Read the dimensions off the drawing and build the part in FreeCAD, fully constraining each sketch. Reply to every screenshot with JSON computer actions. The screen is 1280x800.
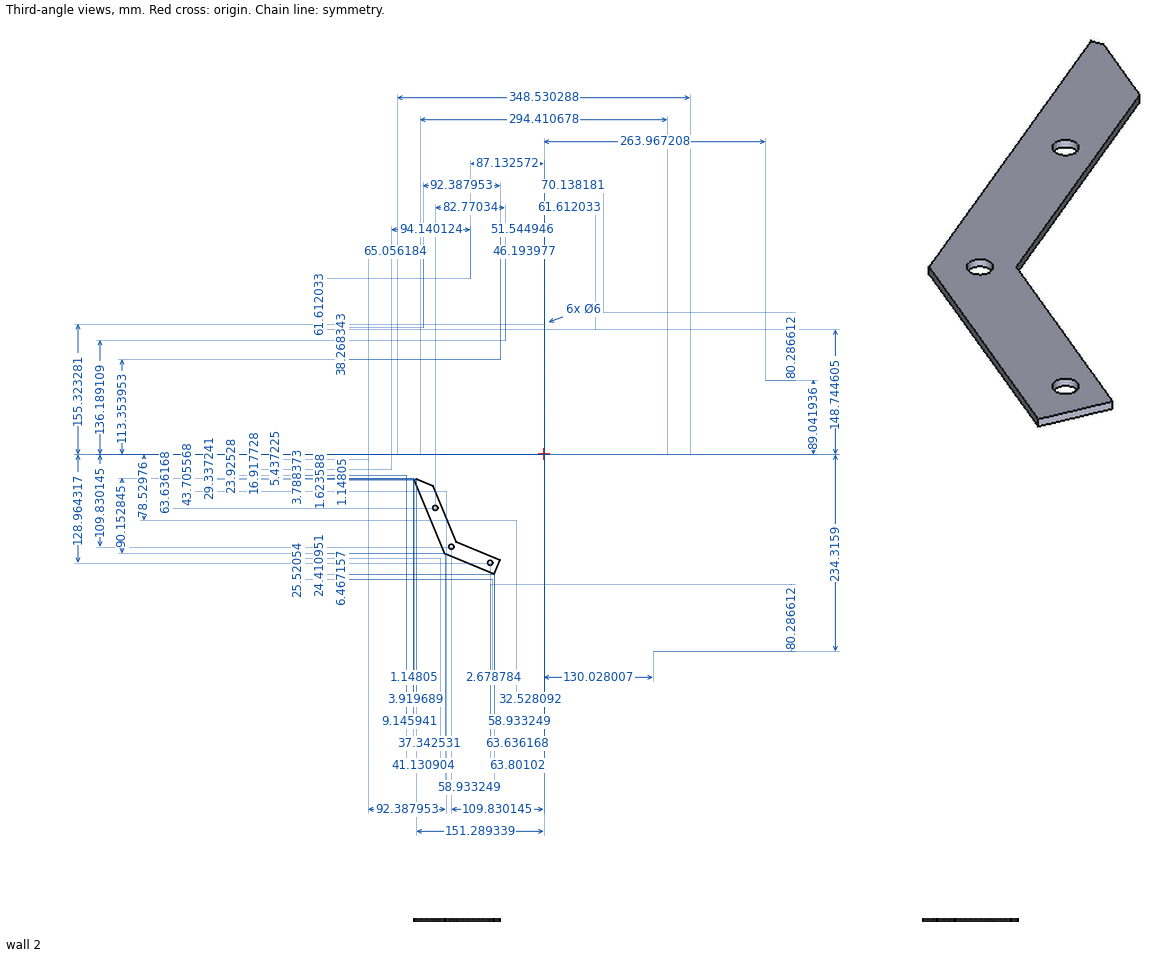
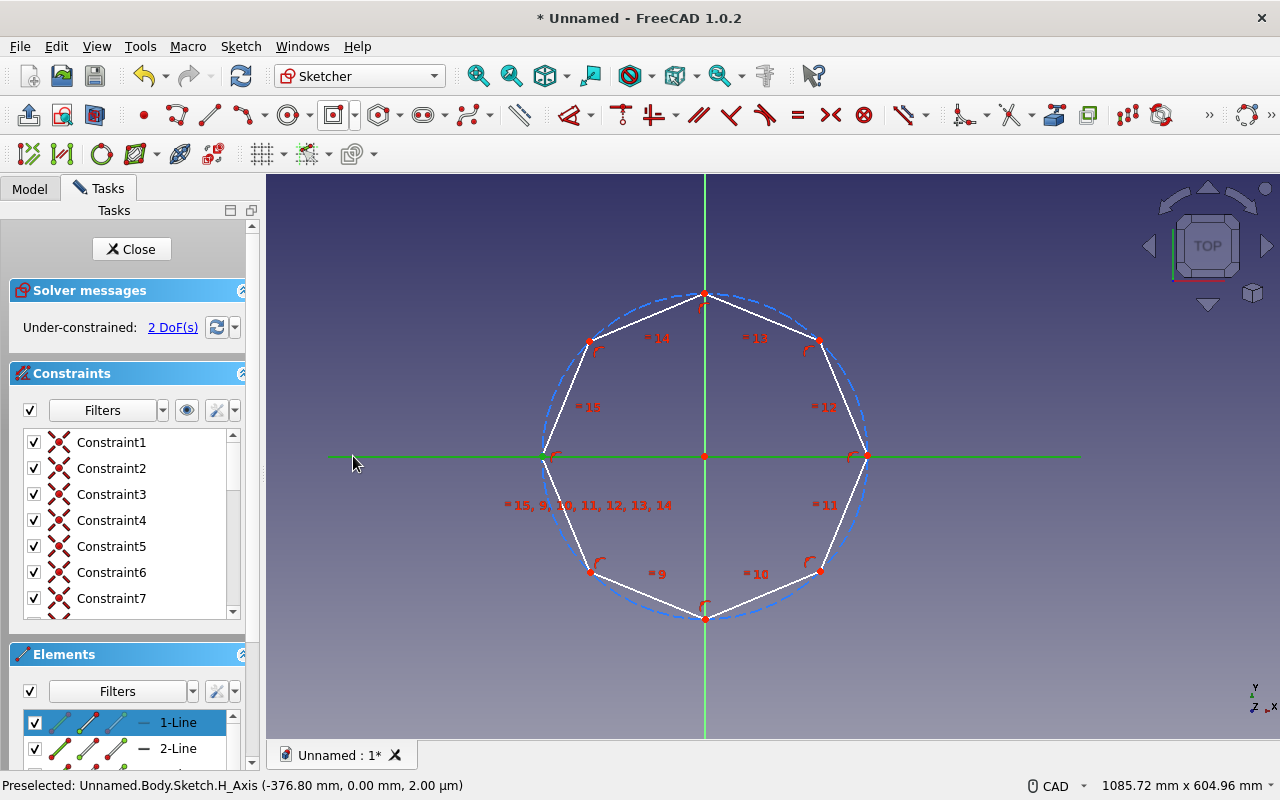
{"action": "left_click", "coordinate": [621, 116]}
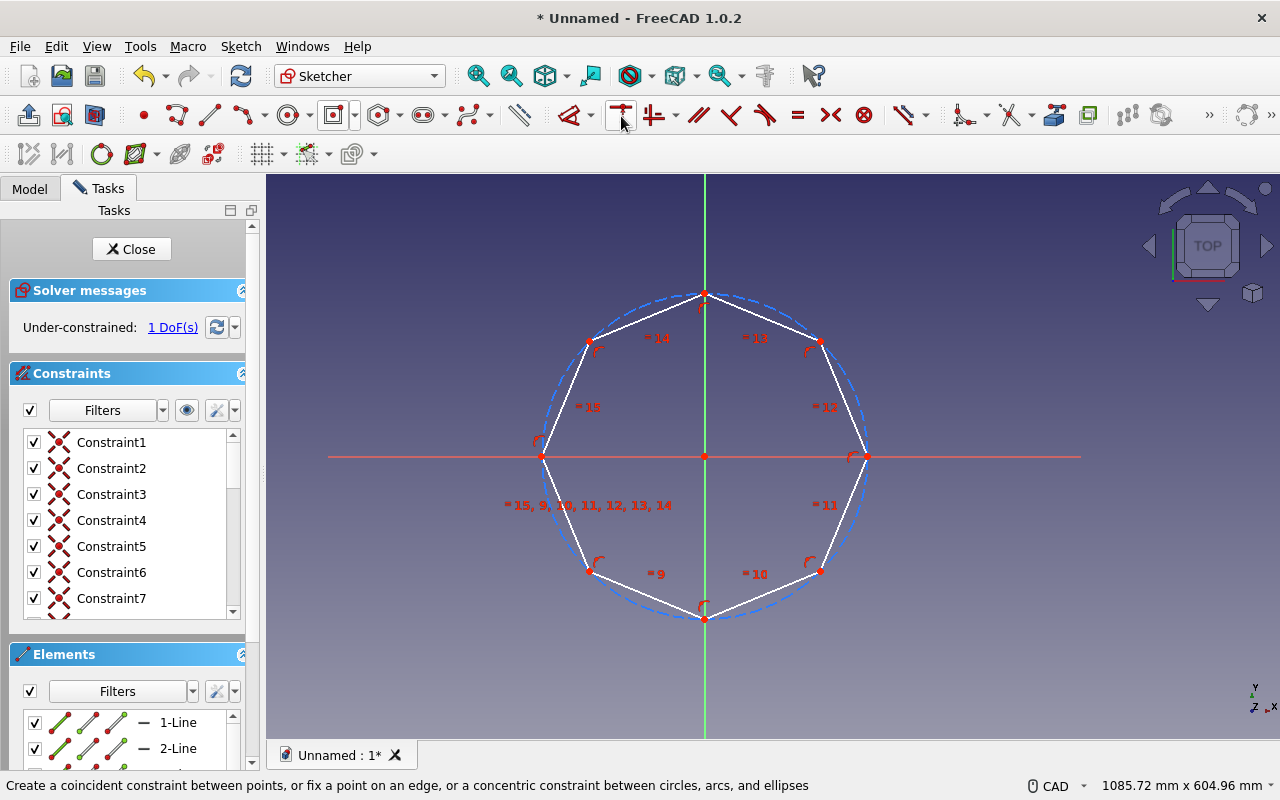
{"action": "left_click", "coordinate": [568, 116]}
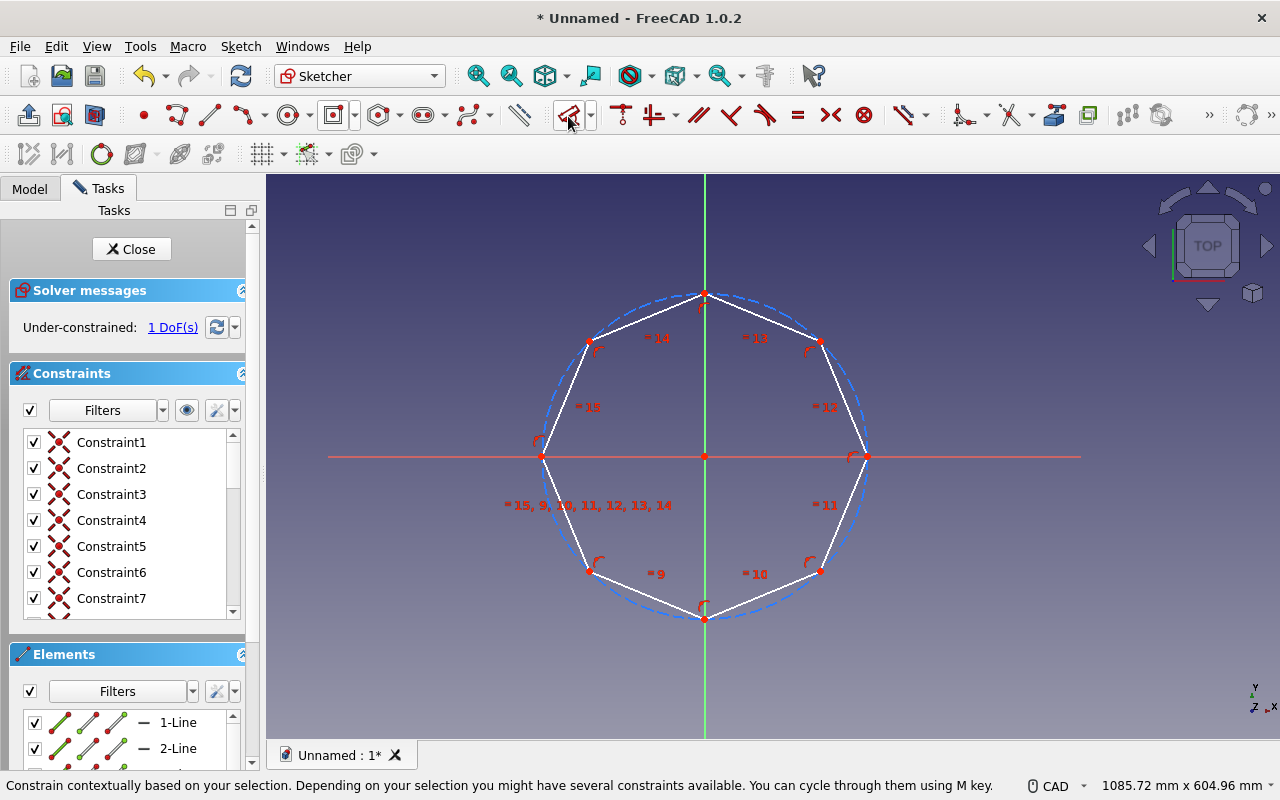
{"action": "left_click", "coordinate": [542, 456]}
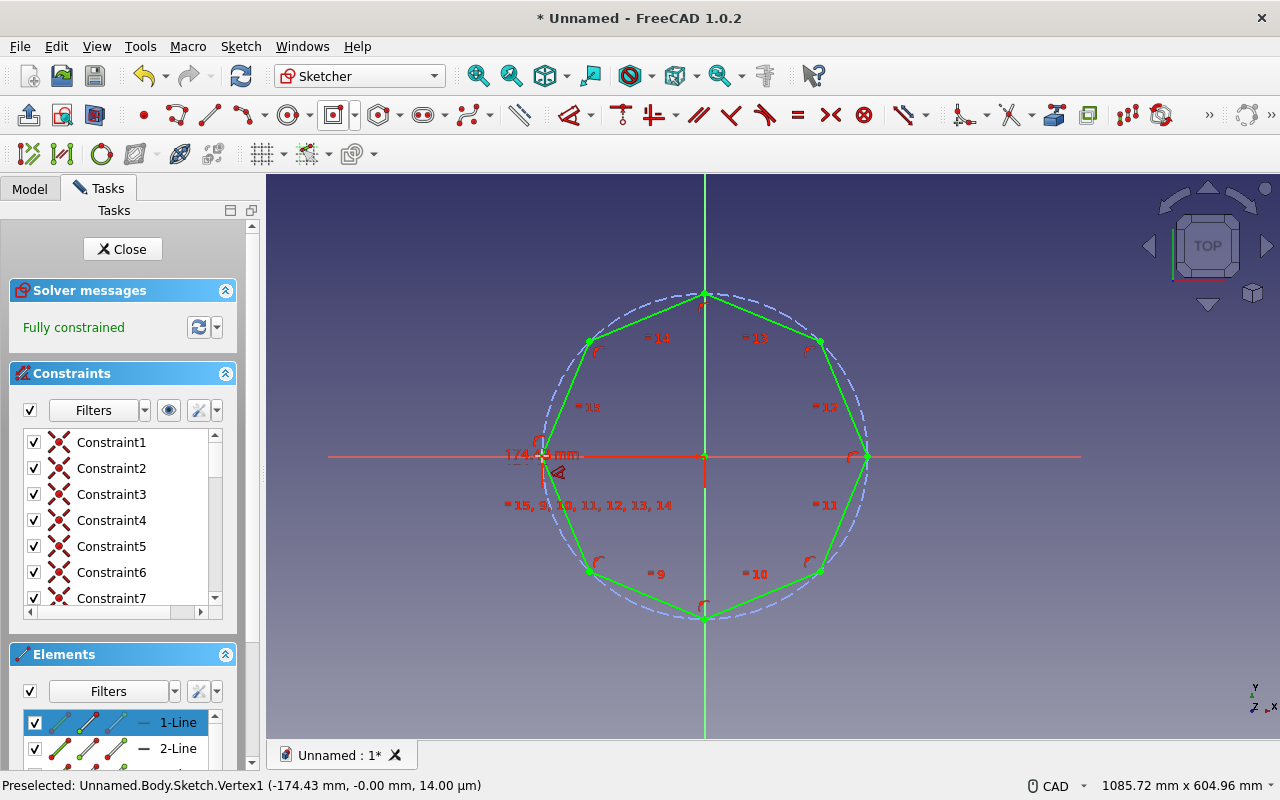
{"action": "left_click", "coordinate": [868, 457]}
{"action": "left_click", "coordinate": [630, 491]}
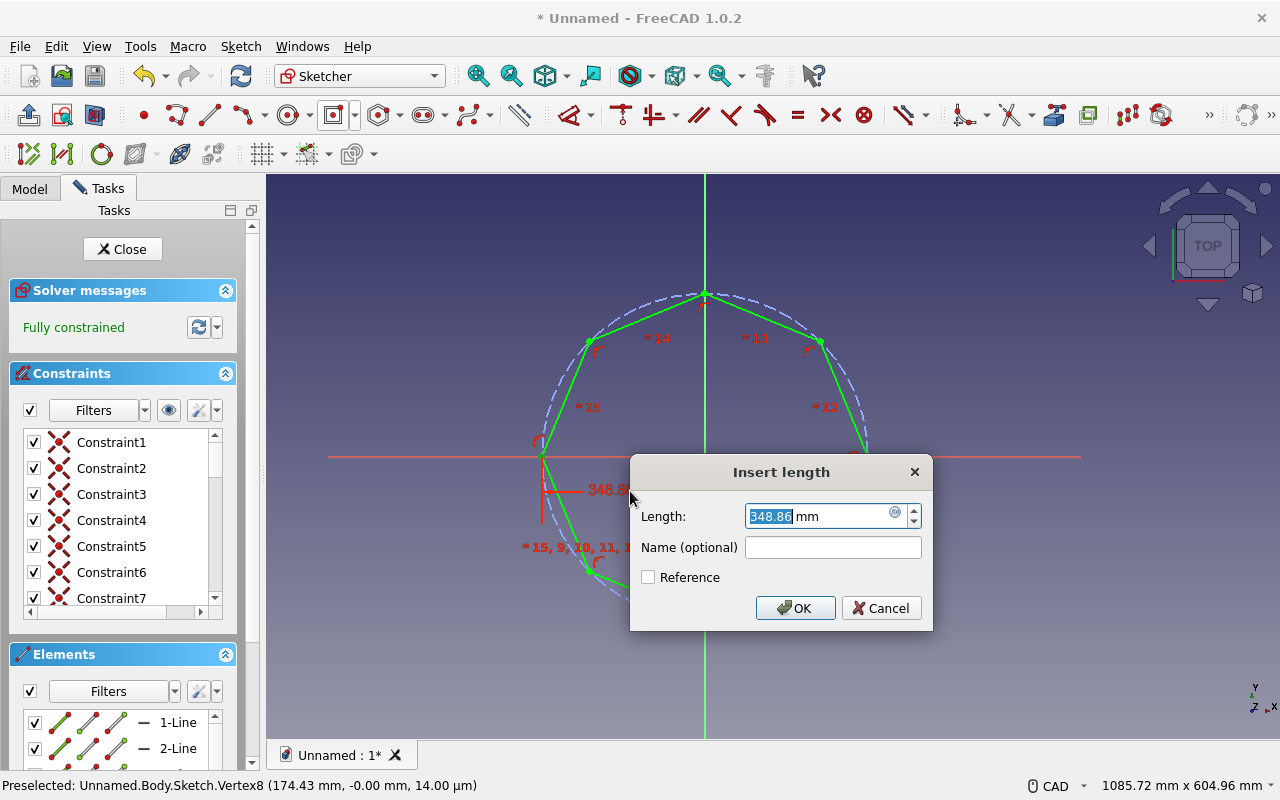
{"action": "type", "text": "348.530288"}
{"action": "key", "text": "Return"}
{"action": "key", "text": "Escape"}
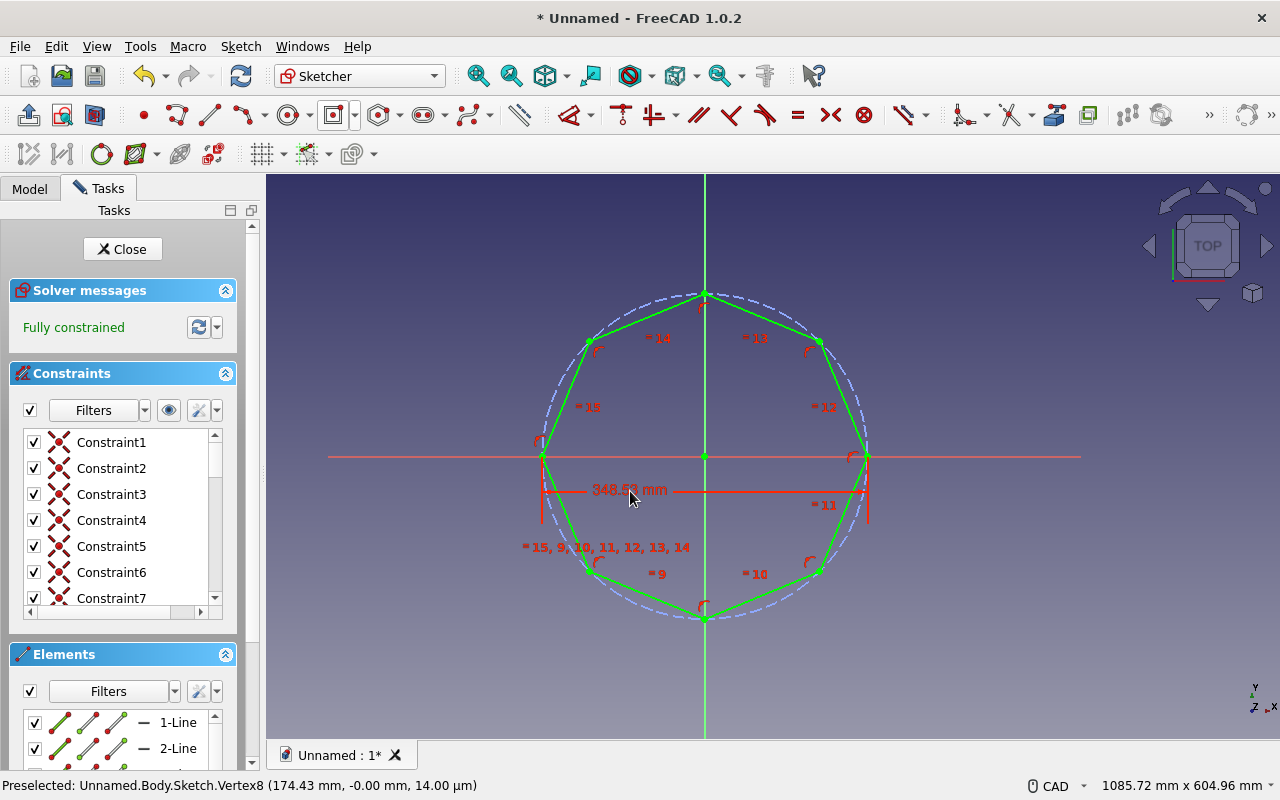
{"action": "left_click", "coordinate": [123, 249]}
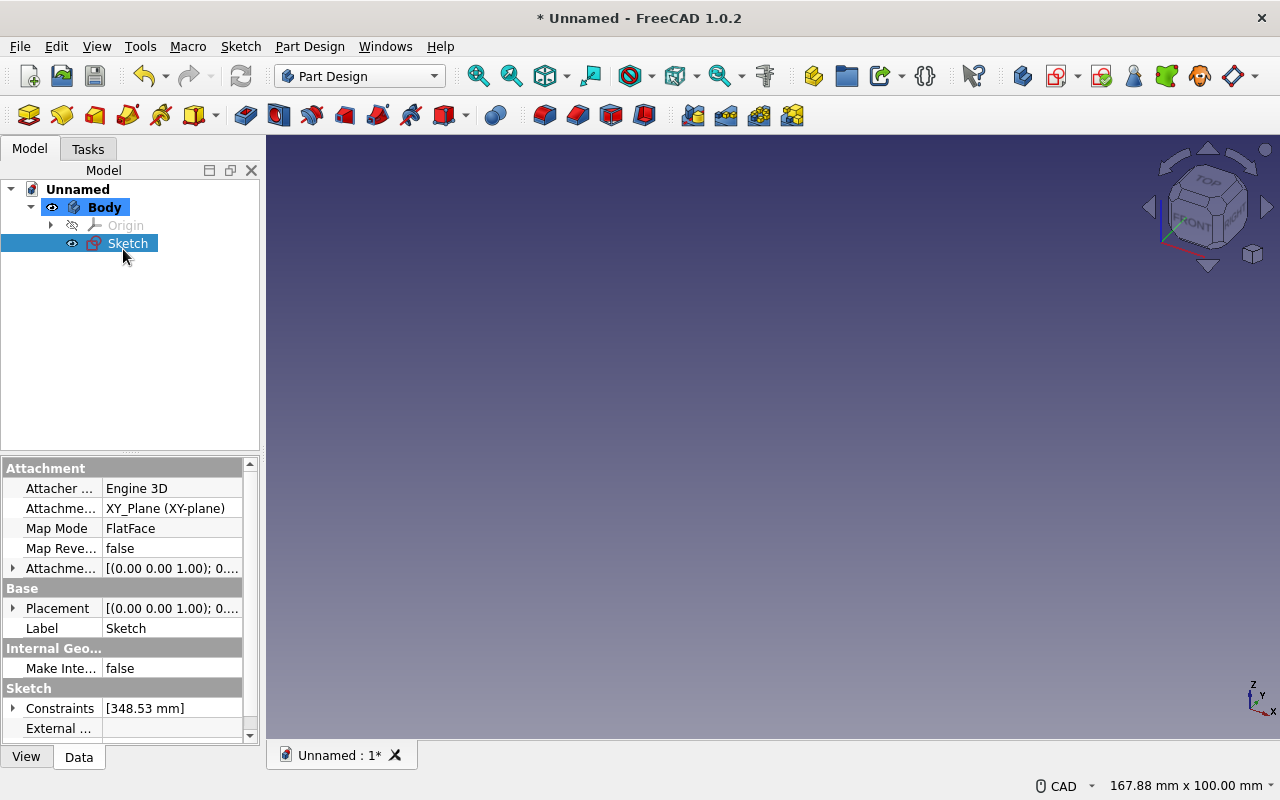
{"action": "left_click", "coordinate": [29, 116]}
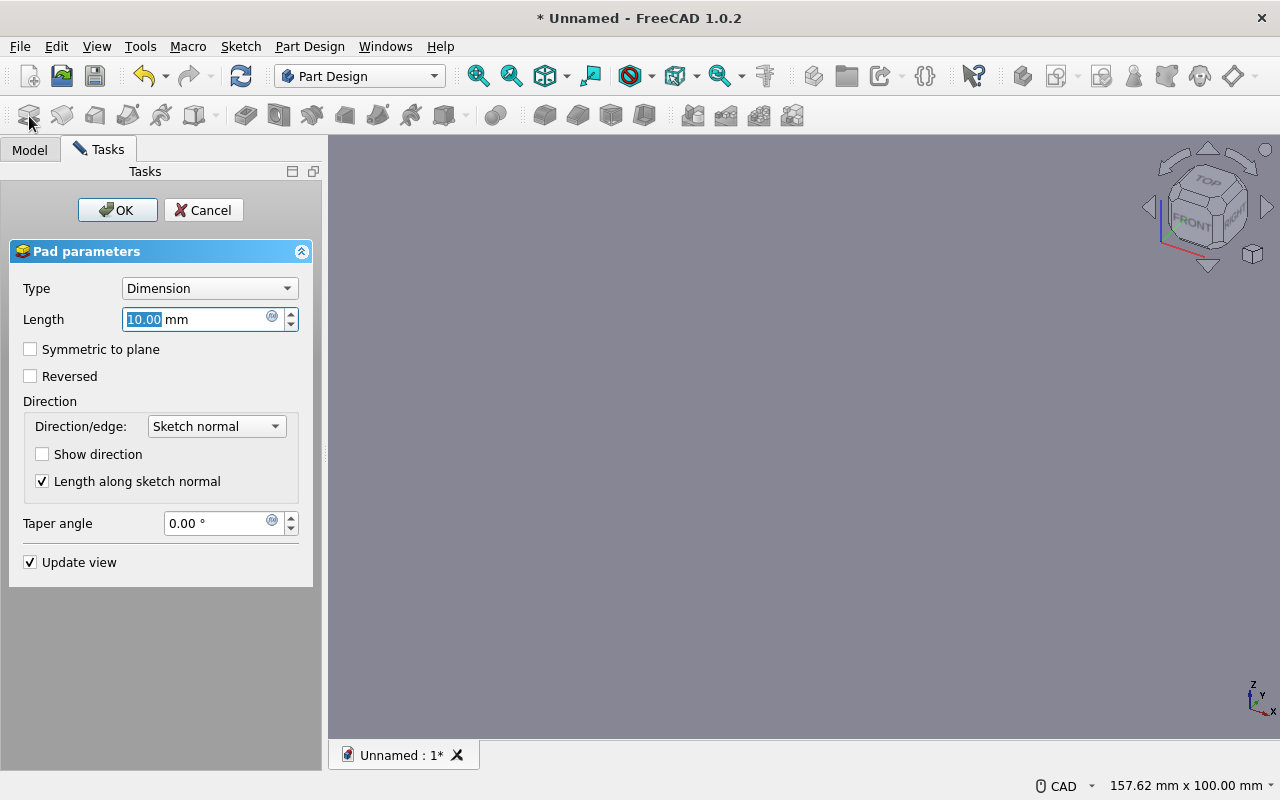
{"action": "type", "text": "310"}
{"action": "key", "text": "Tab"}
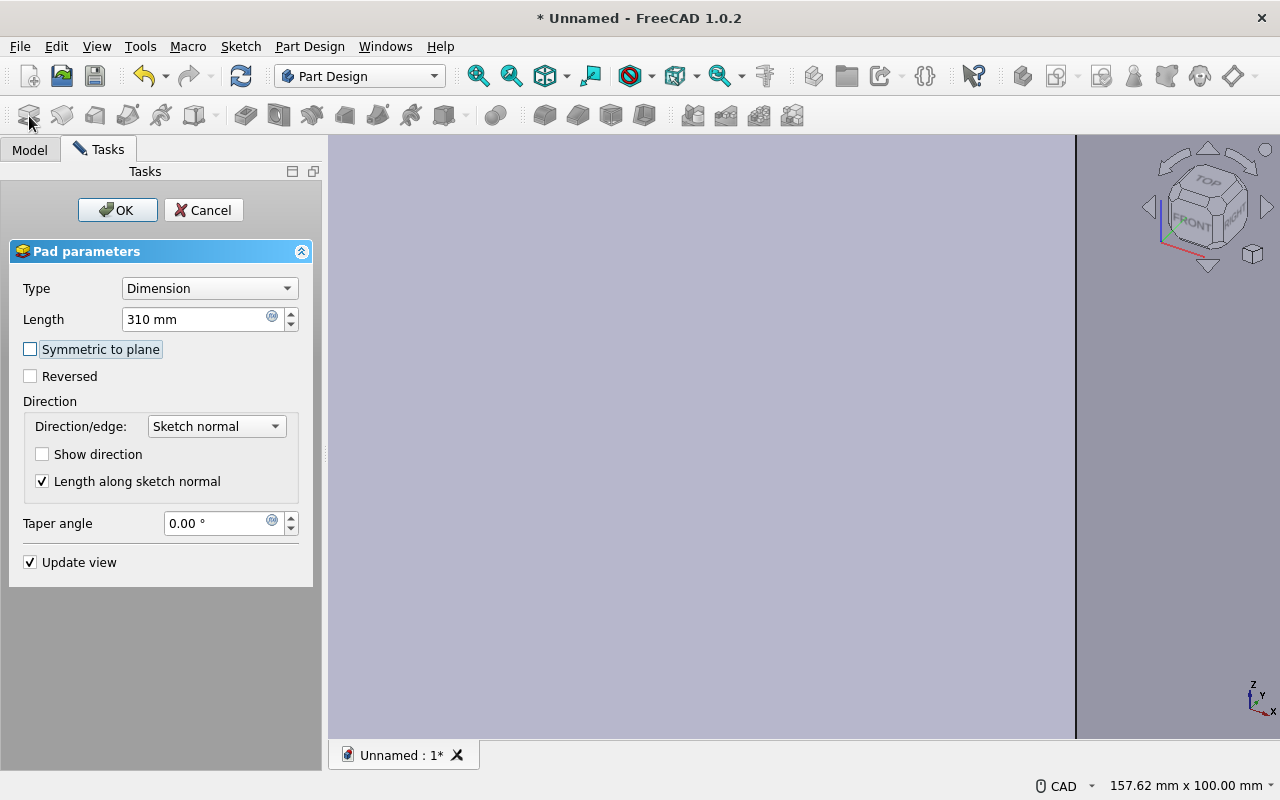
{"action": "left_click", "coordinate": [118, 210]}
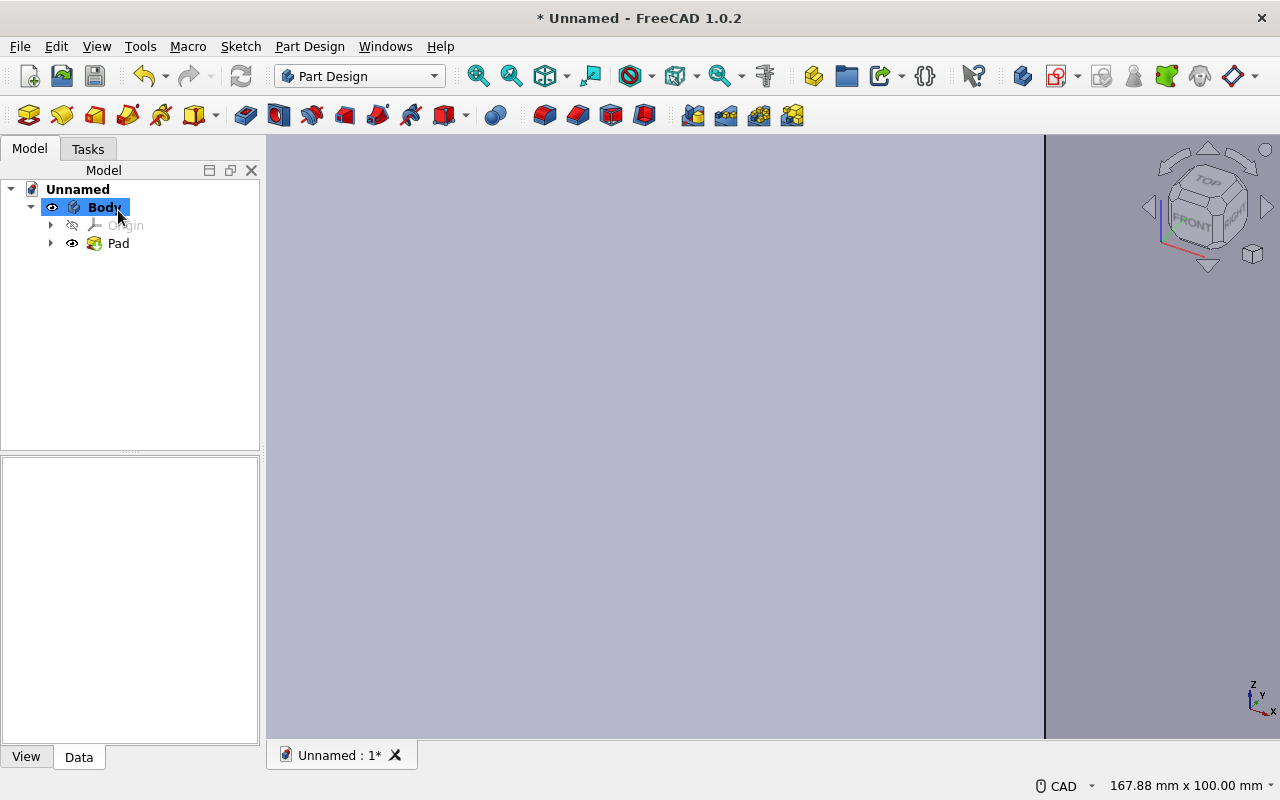
{"action": "left_click", "coordinate": [479, 76]}